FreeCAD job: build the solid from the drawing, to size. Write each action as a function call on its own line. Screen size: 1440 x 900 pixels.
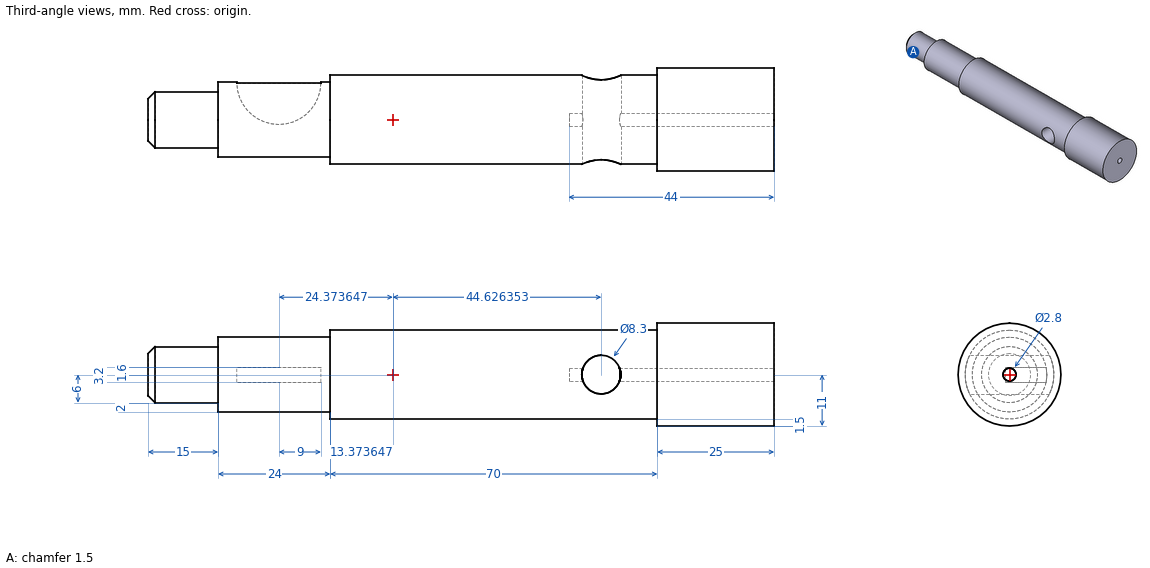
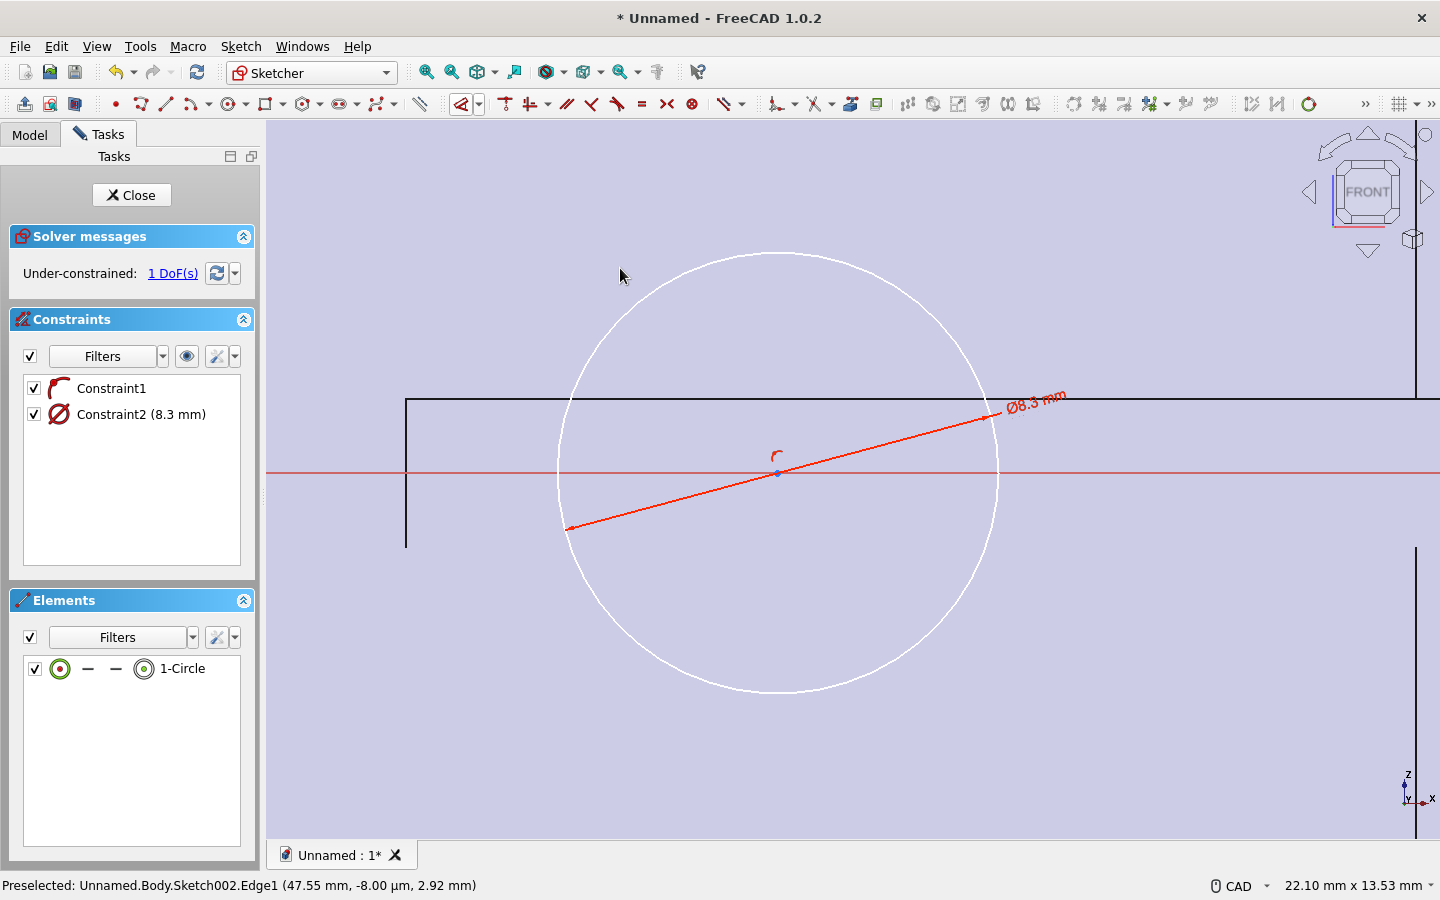
click(778, 473)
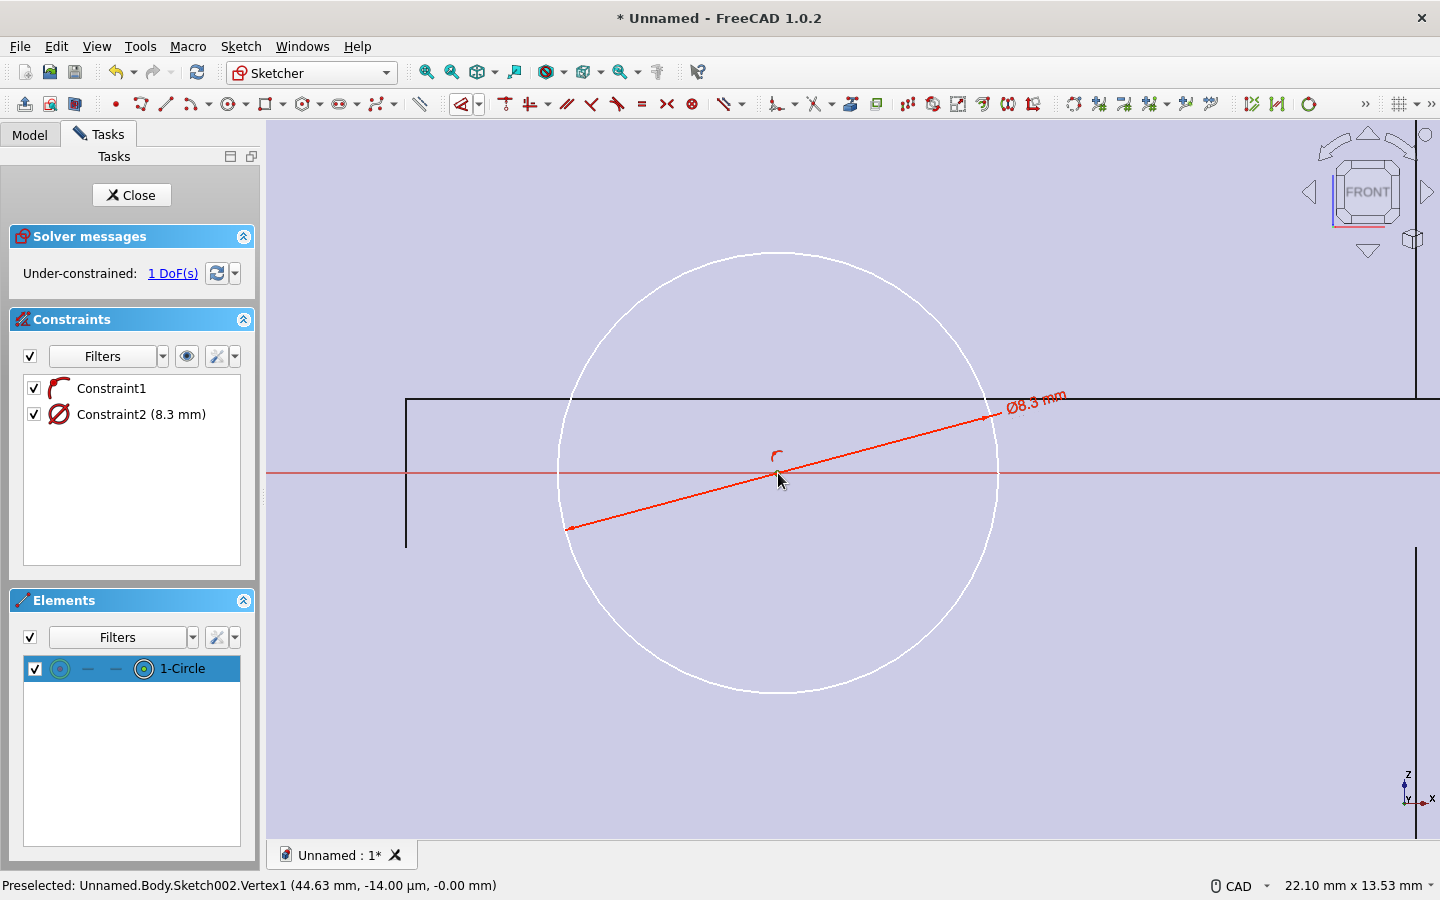
click(478, 104)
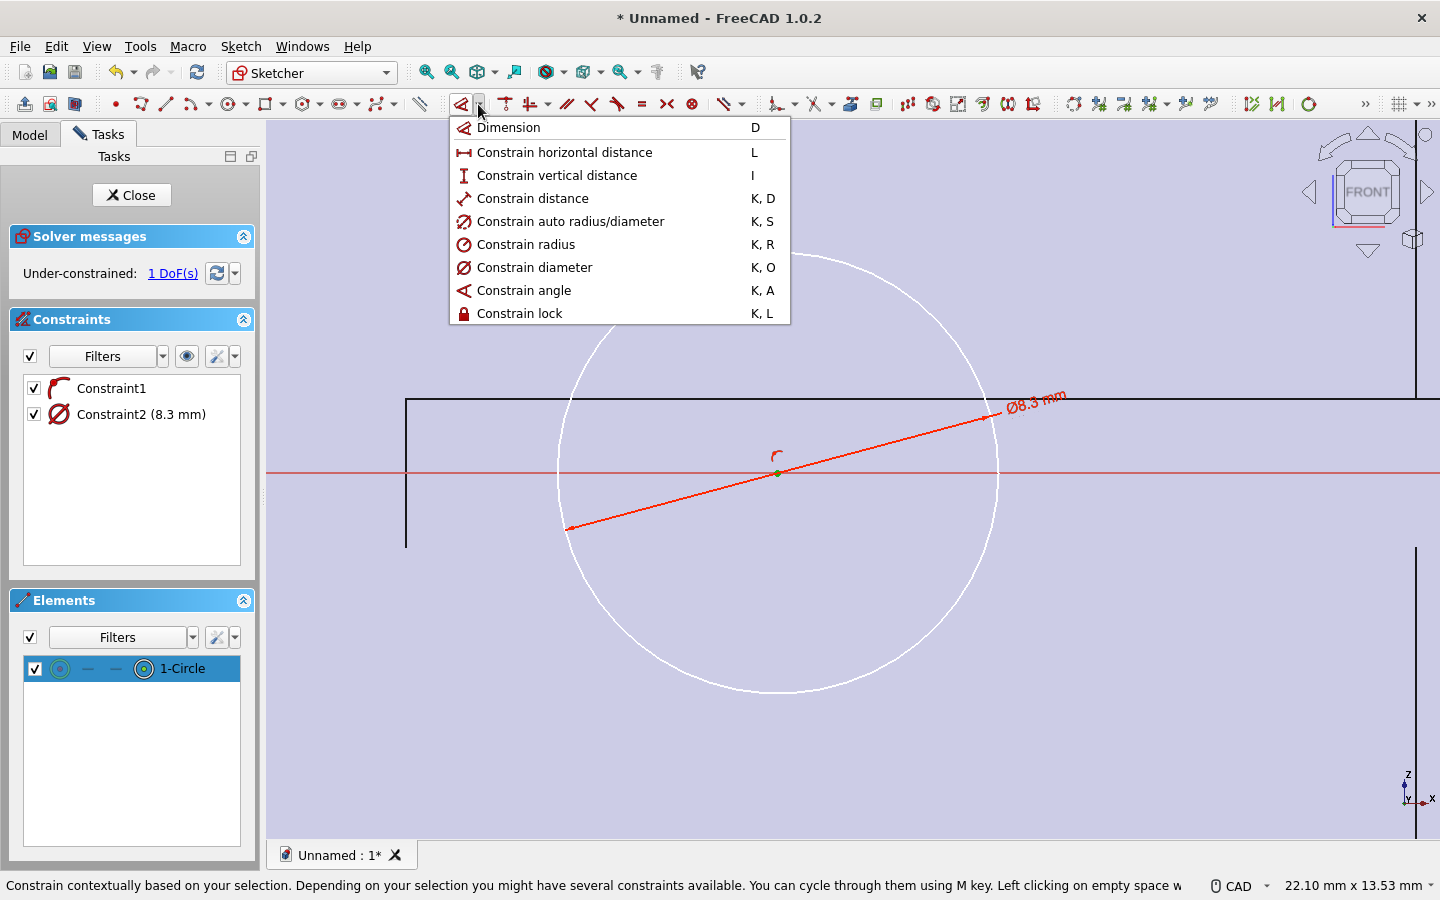
click(620, 152)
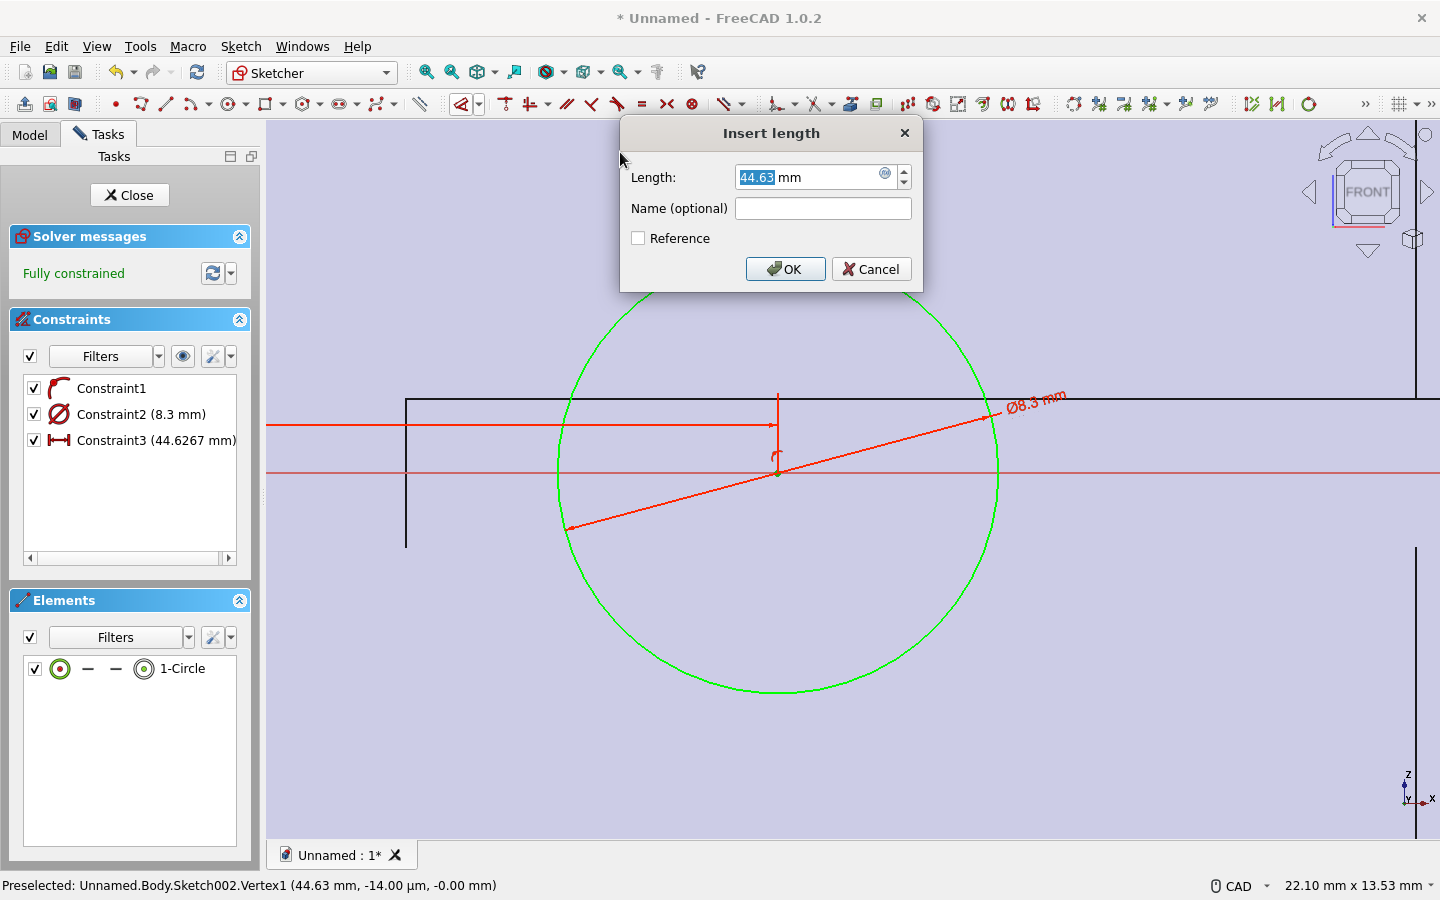
text(44.626353)
key(Return)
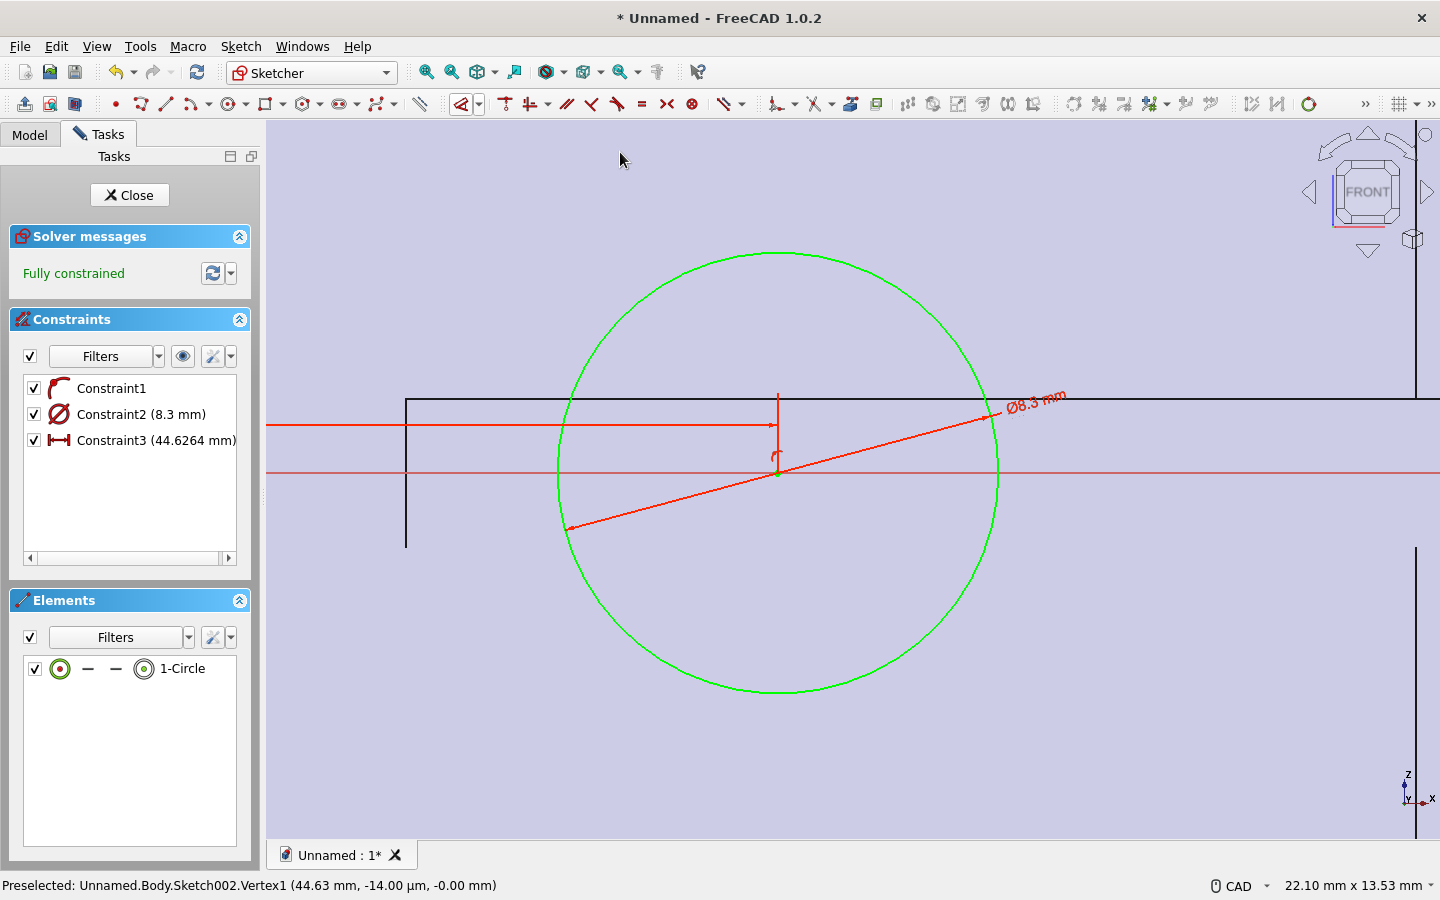
click(130, 195)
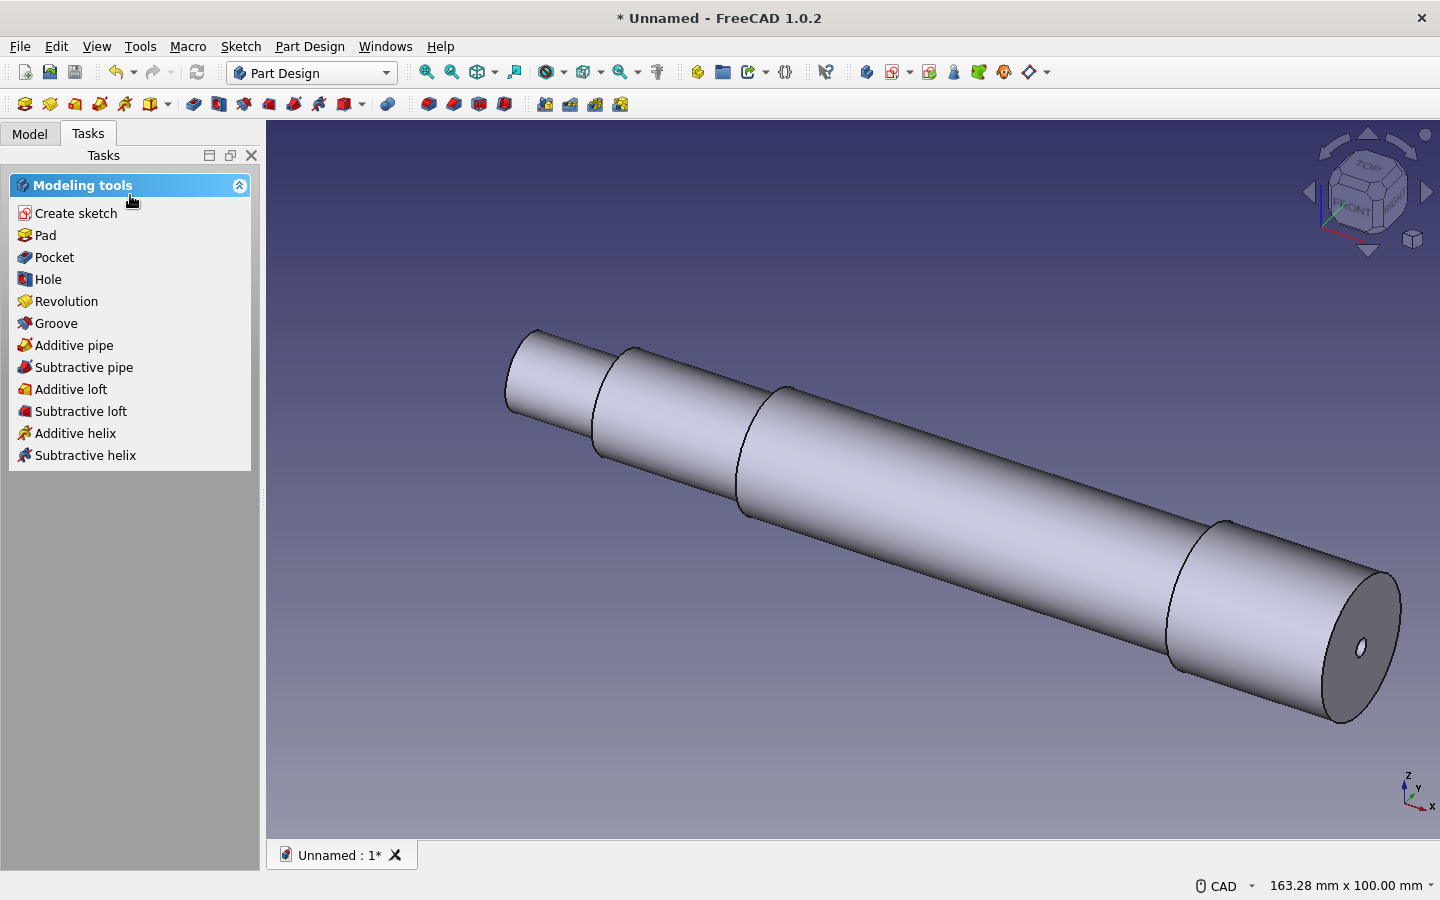
click(194, 104)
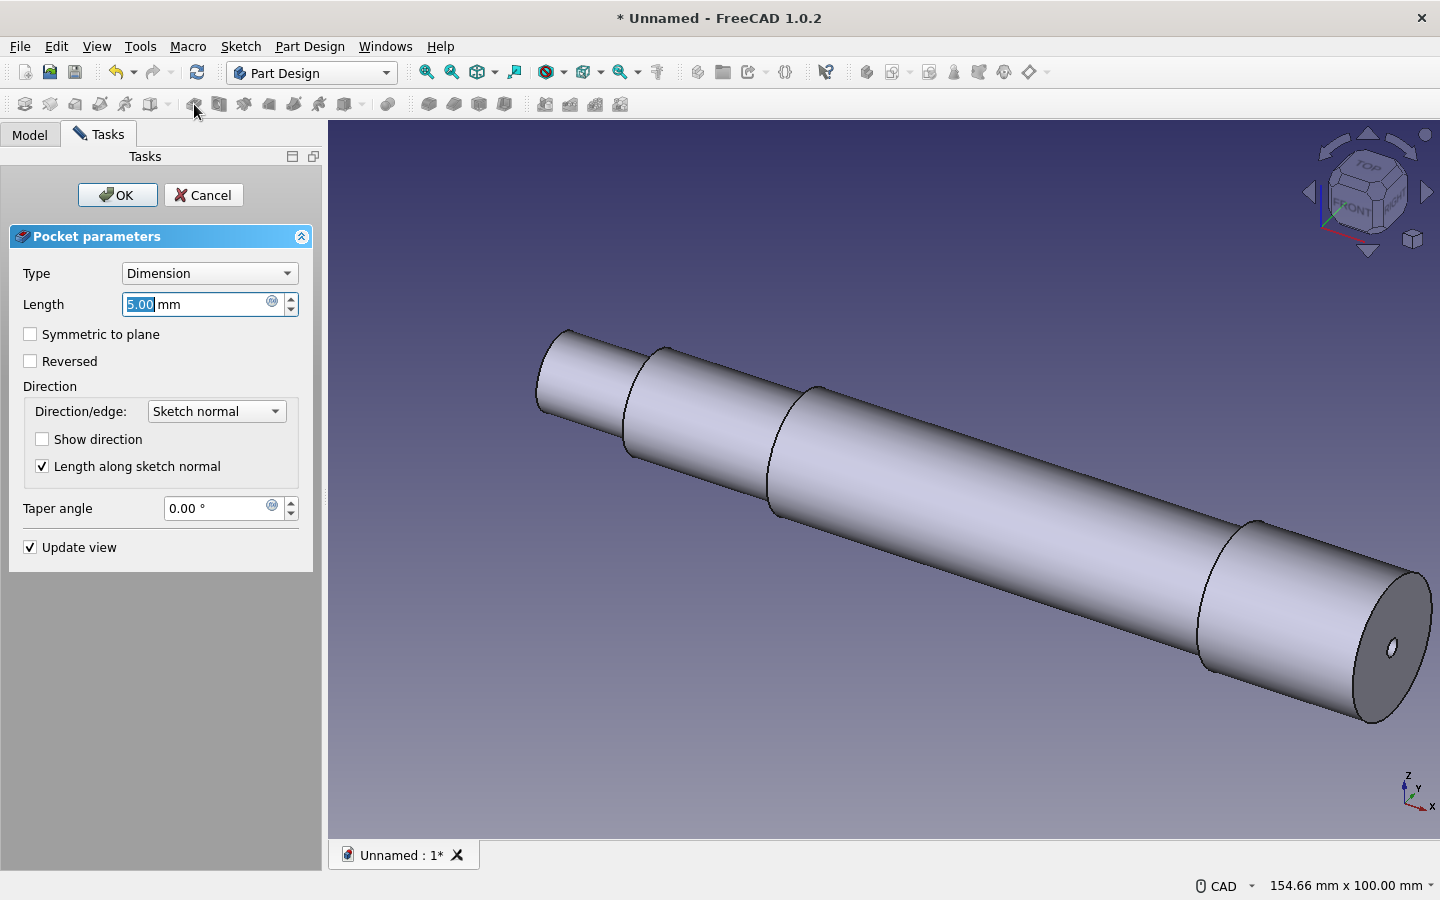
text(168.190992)
key(Tab)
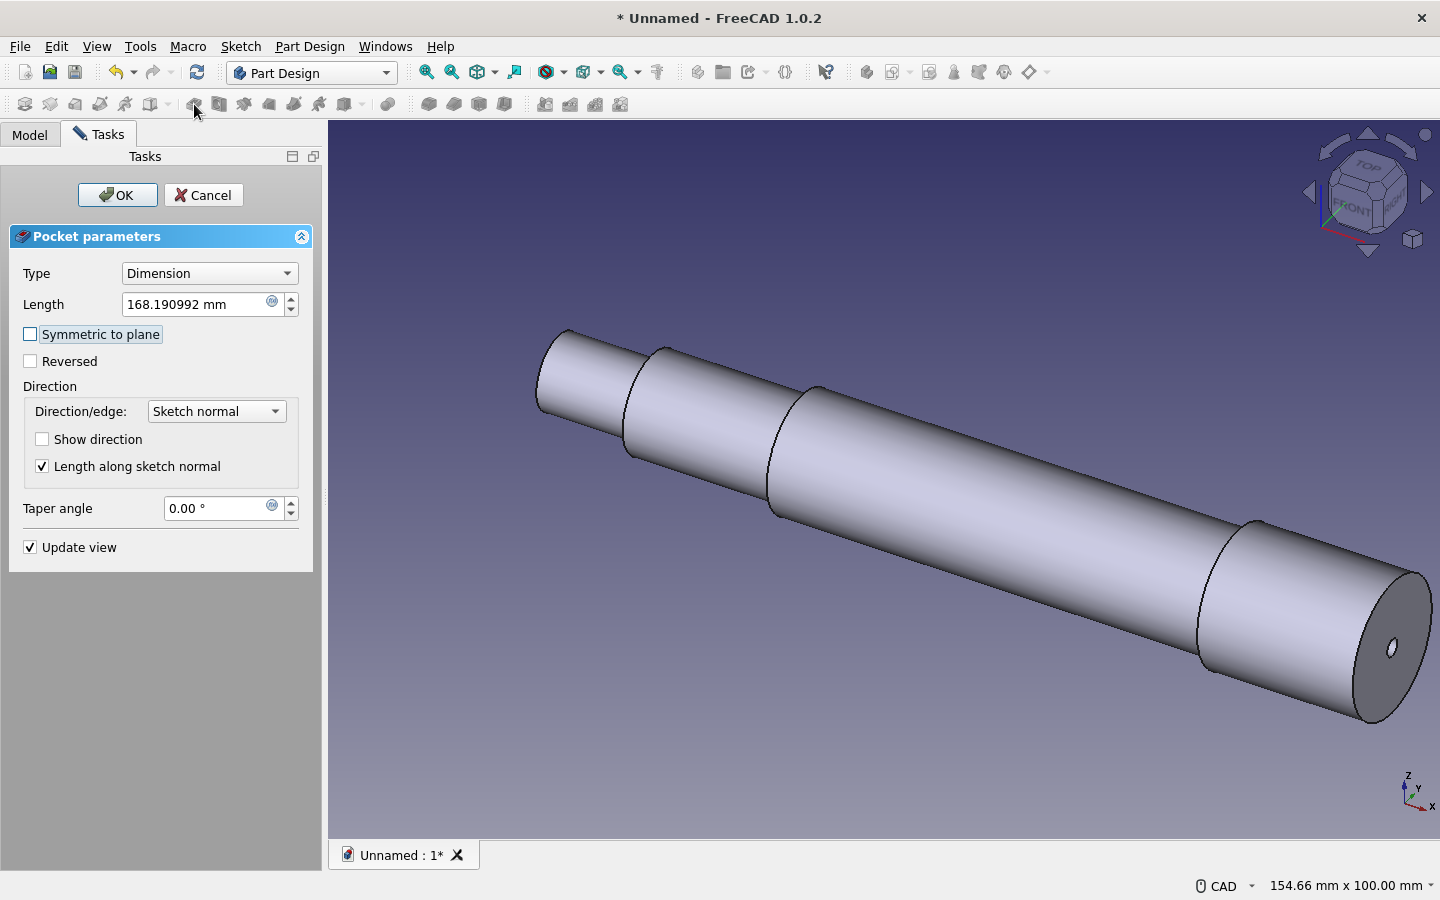
click(31, 334)